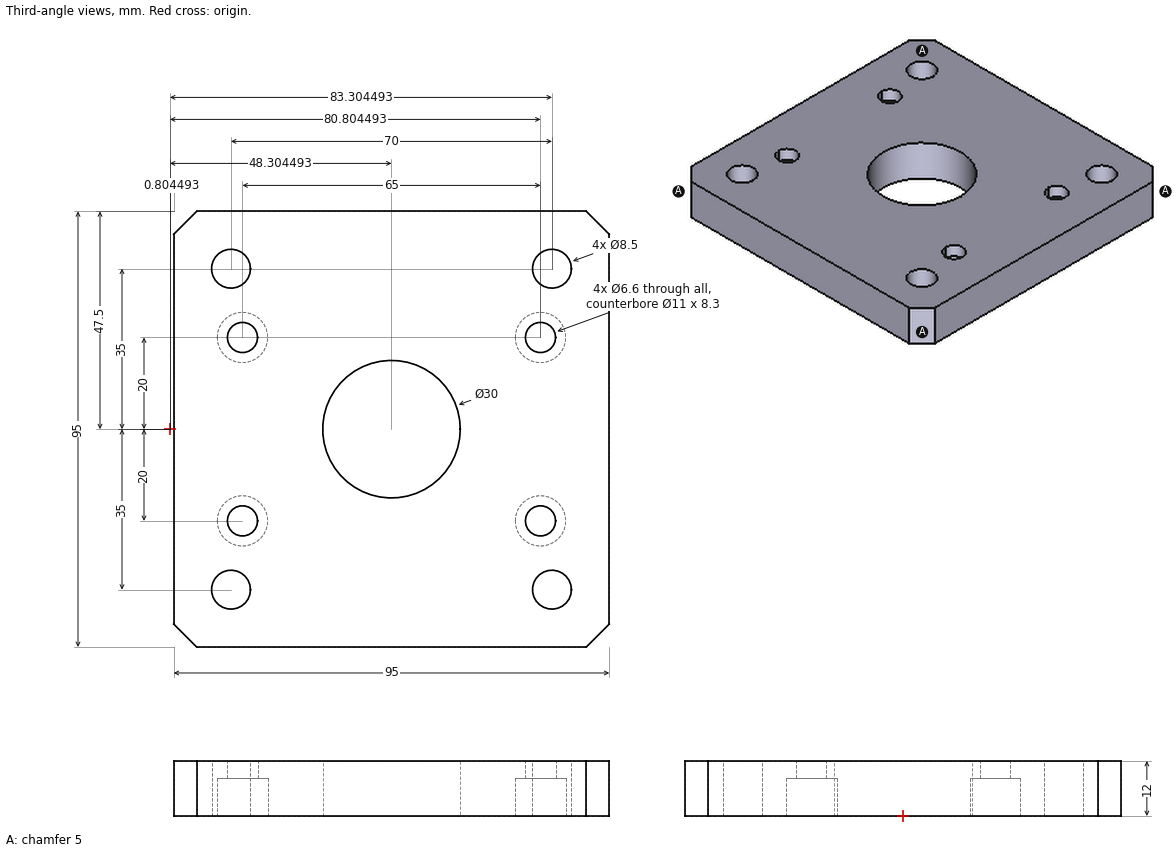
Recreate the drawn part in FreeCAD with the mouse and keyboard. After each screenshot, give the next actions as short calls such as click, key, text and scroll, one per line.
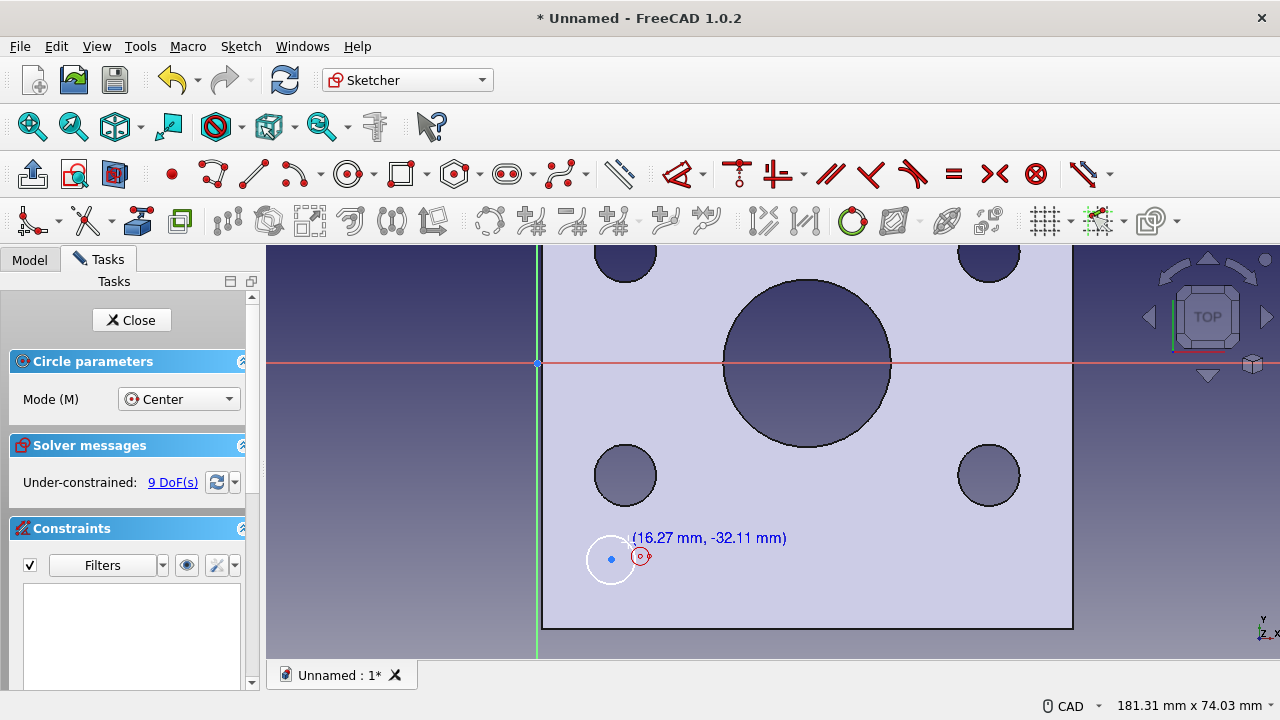
click(1003, 559)
click(1020, 542)
key(Escape)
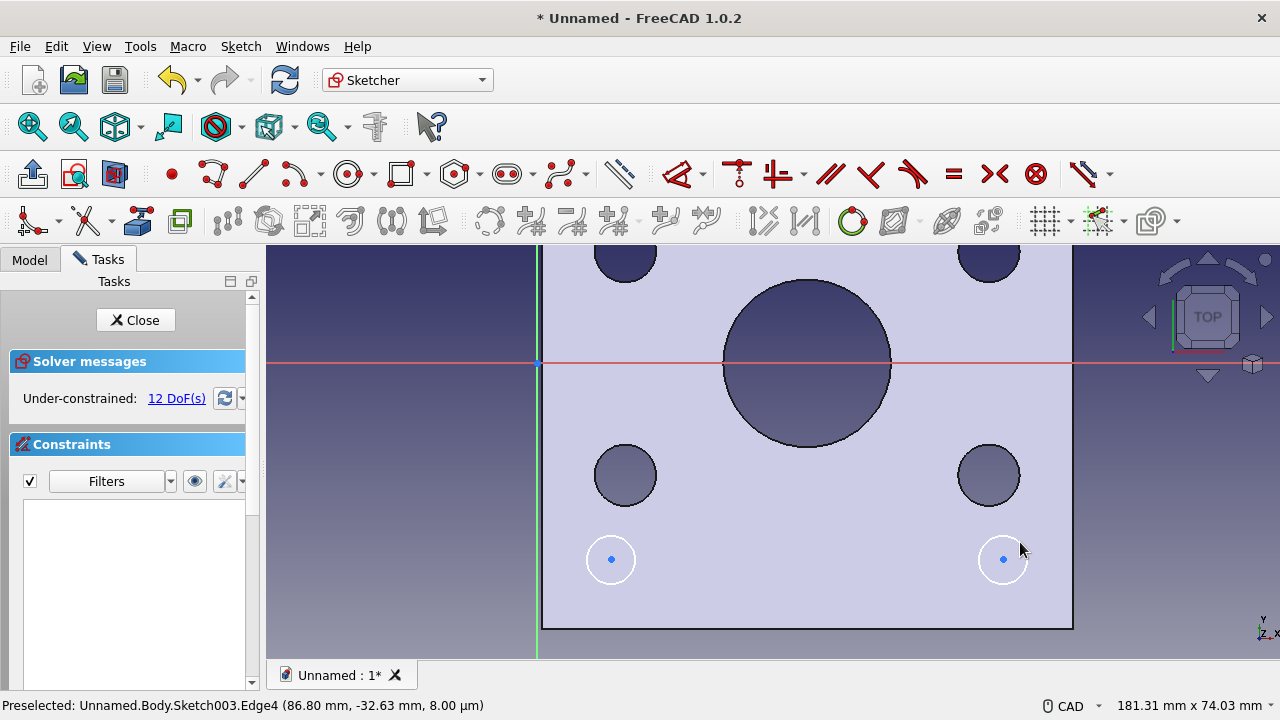
scroll(610, 560, down, 3)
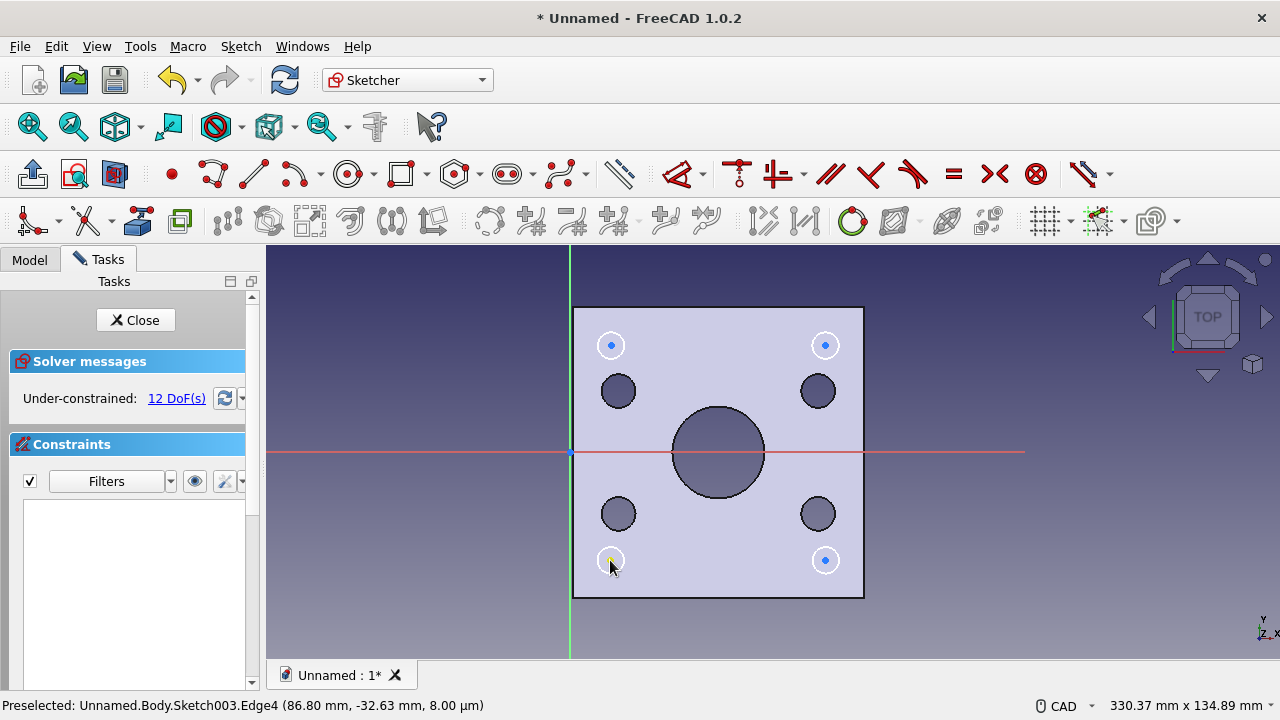
click(835, 336)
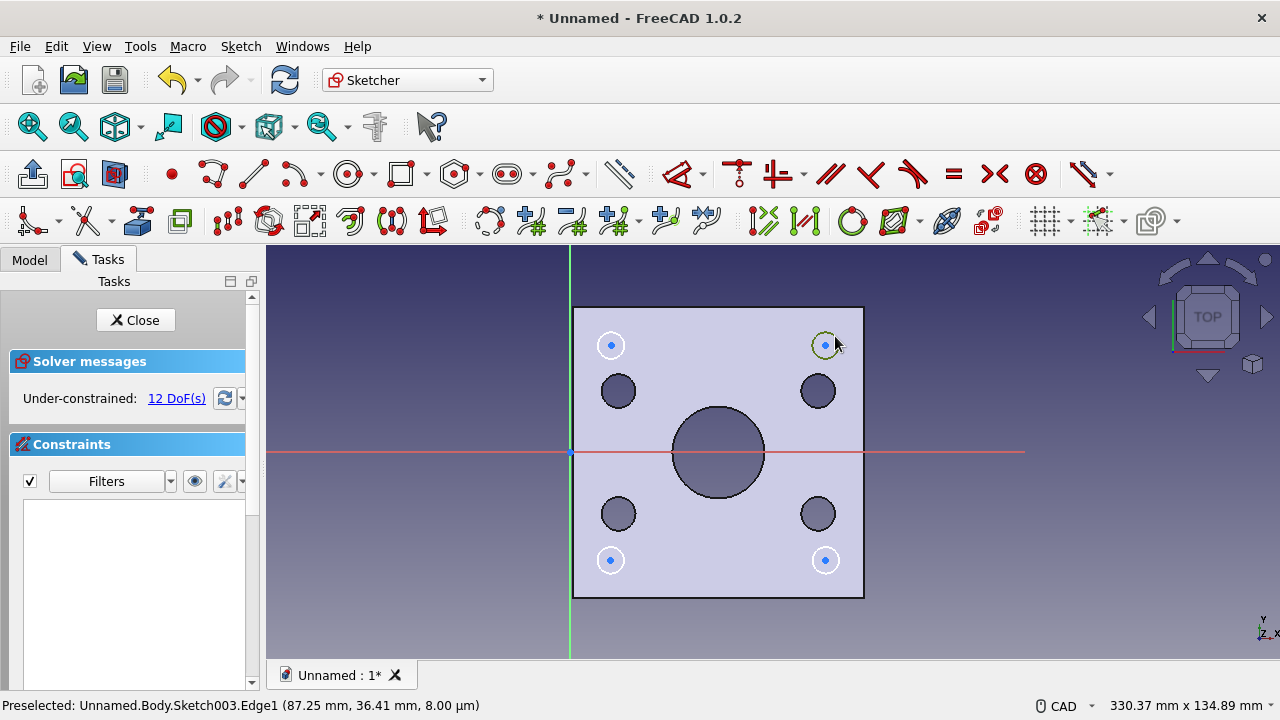
click(620, 336)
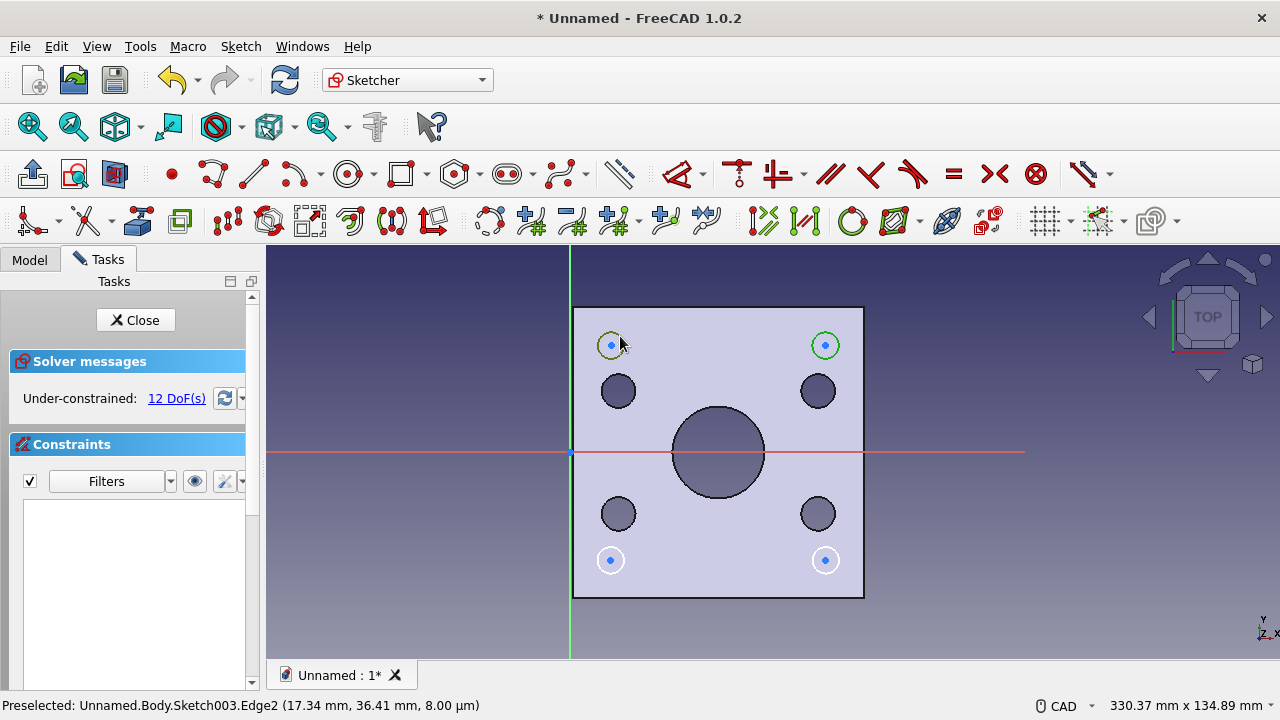
click(620, 551)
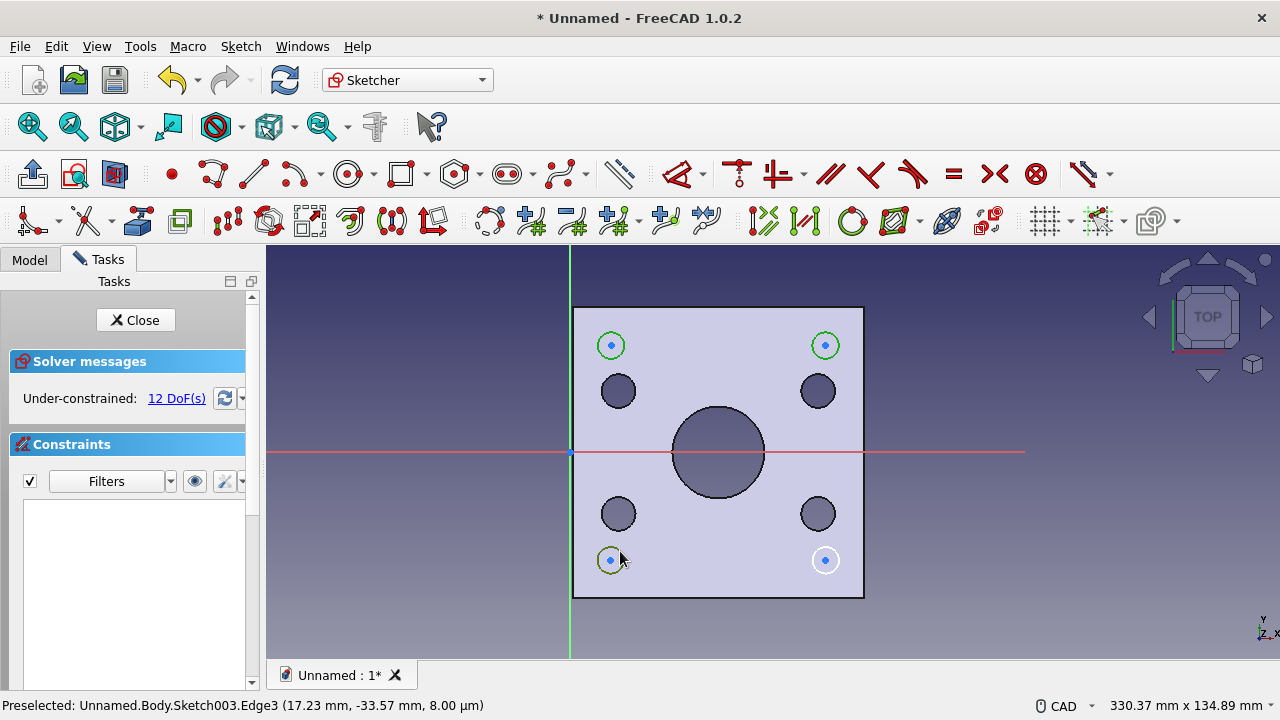
click(835, 551)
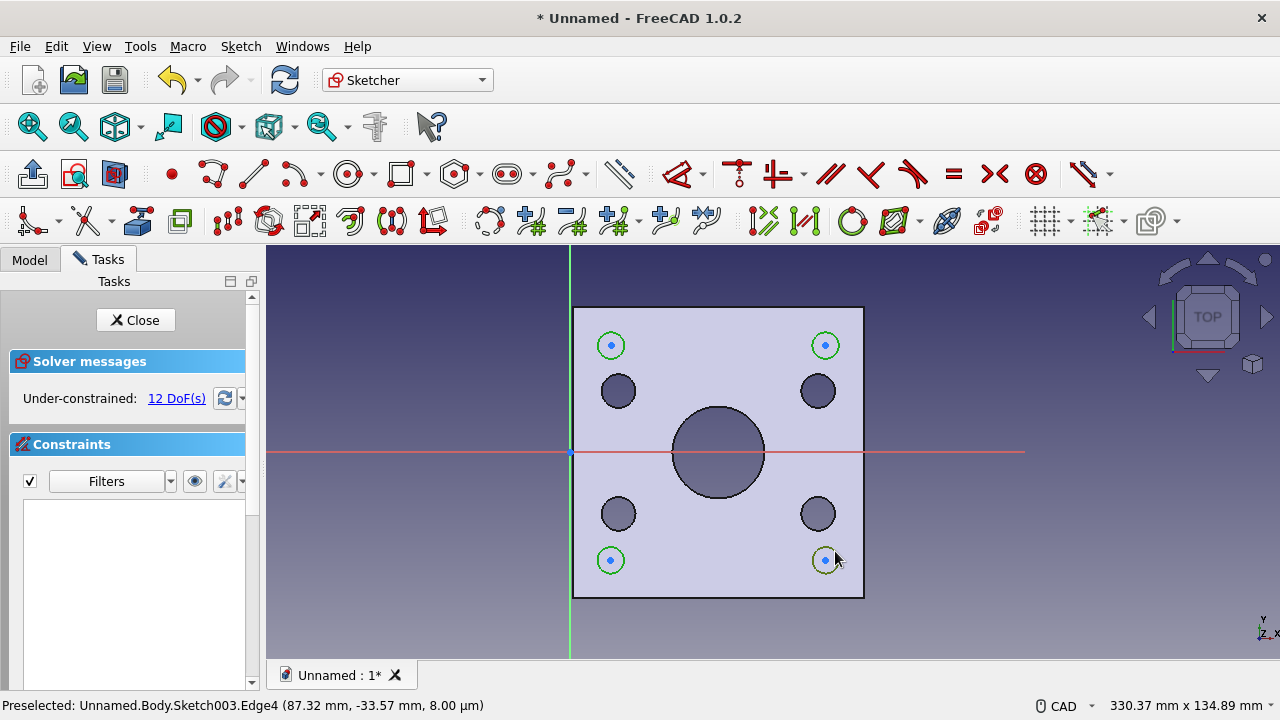
click(954, 174)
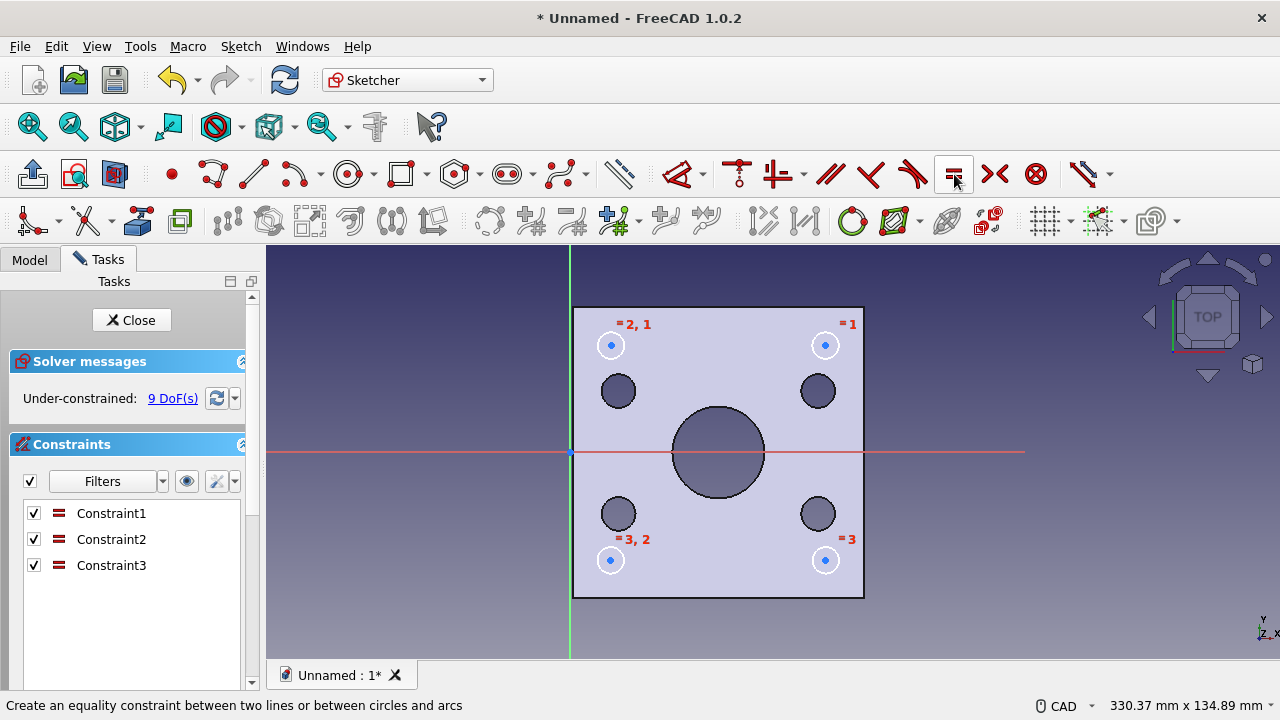
click(826, 346)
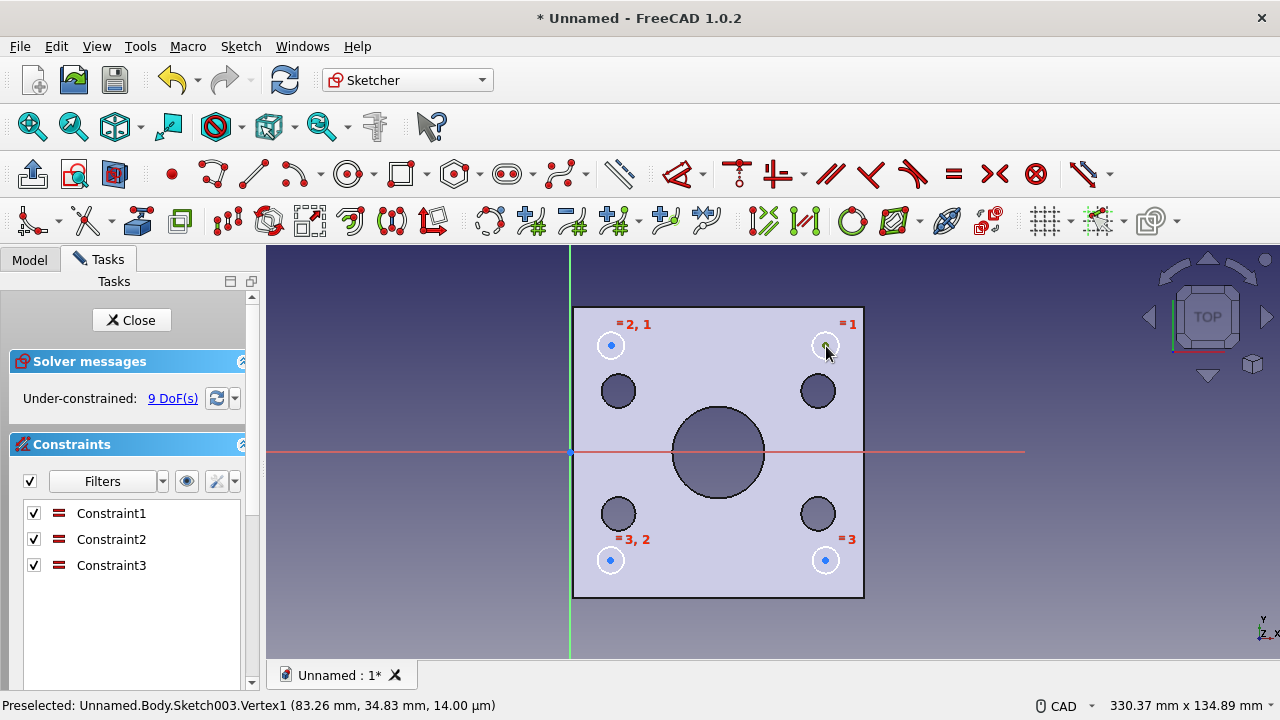
click(611, 346)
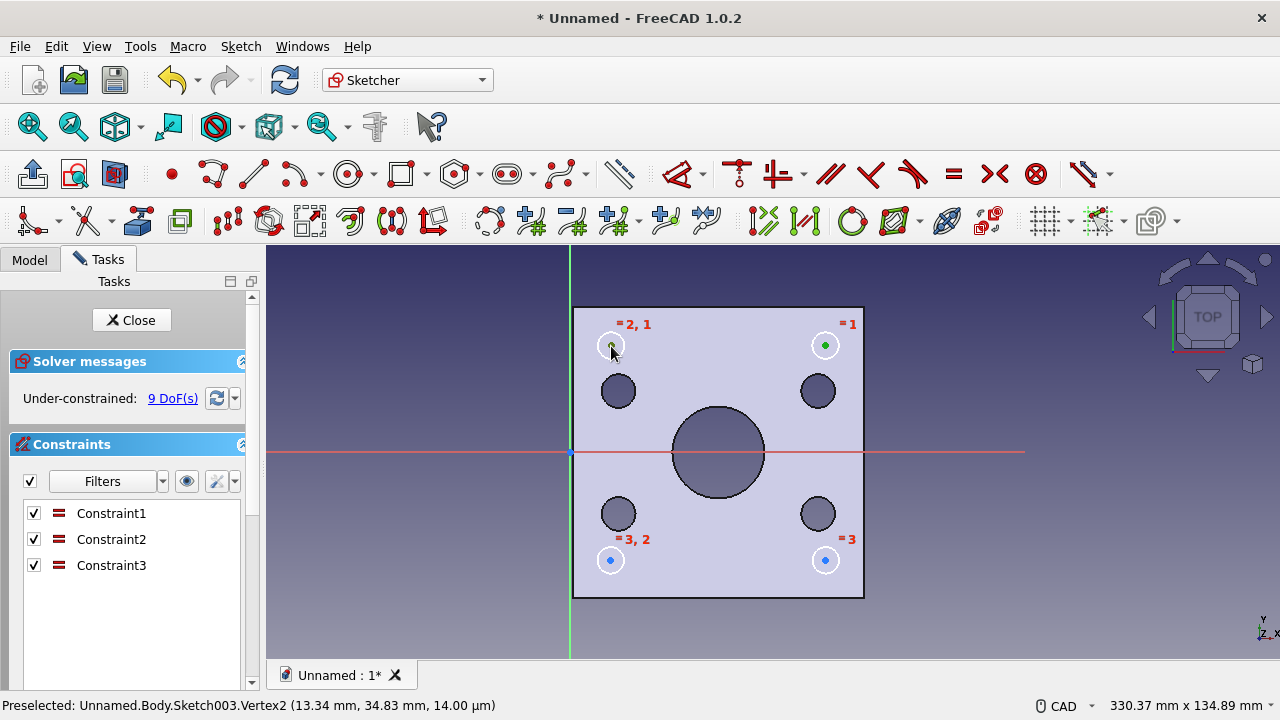
click(804, 174)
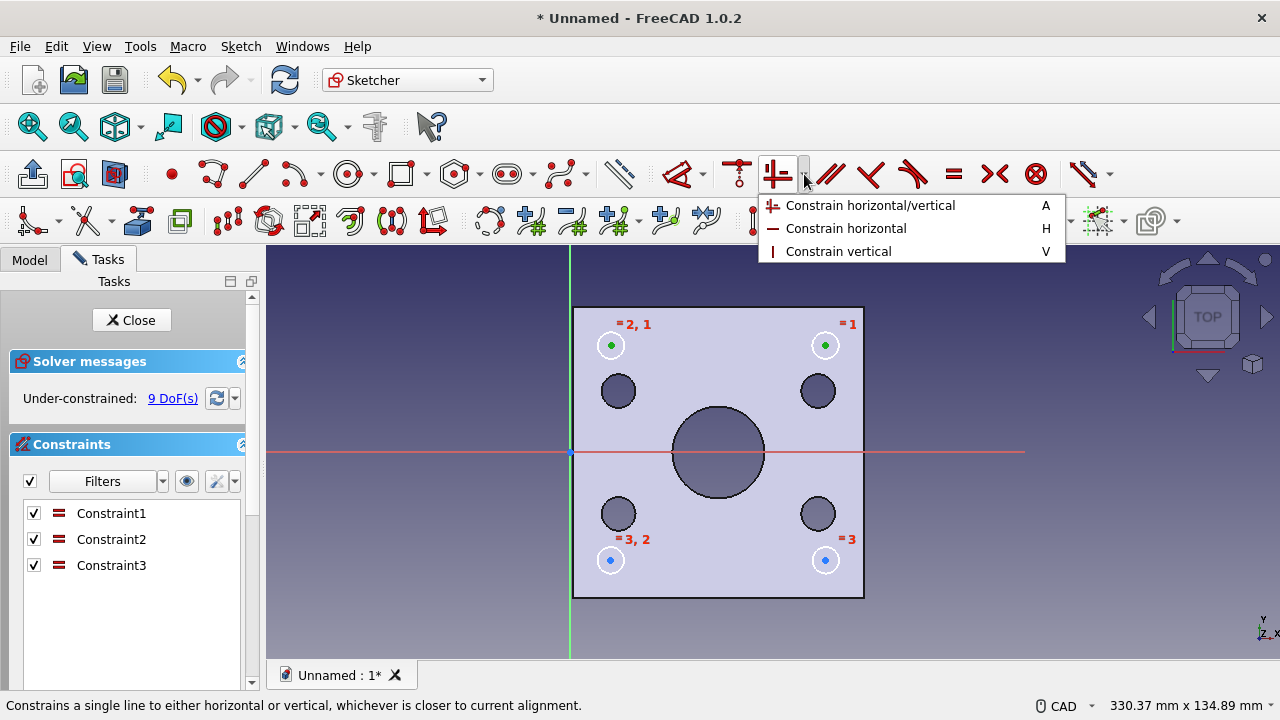
click(912, 228)